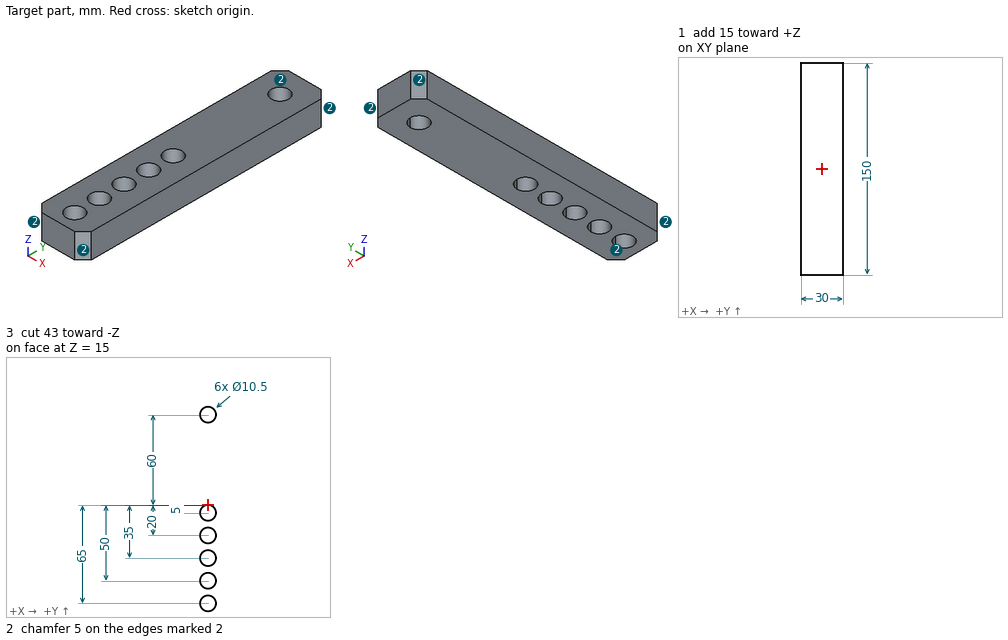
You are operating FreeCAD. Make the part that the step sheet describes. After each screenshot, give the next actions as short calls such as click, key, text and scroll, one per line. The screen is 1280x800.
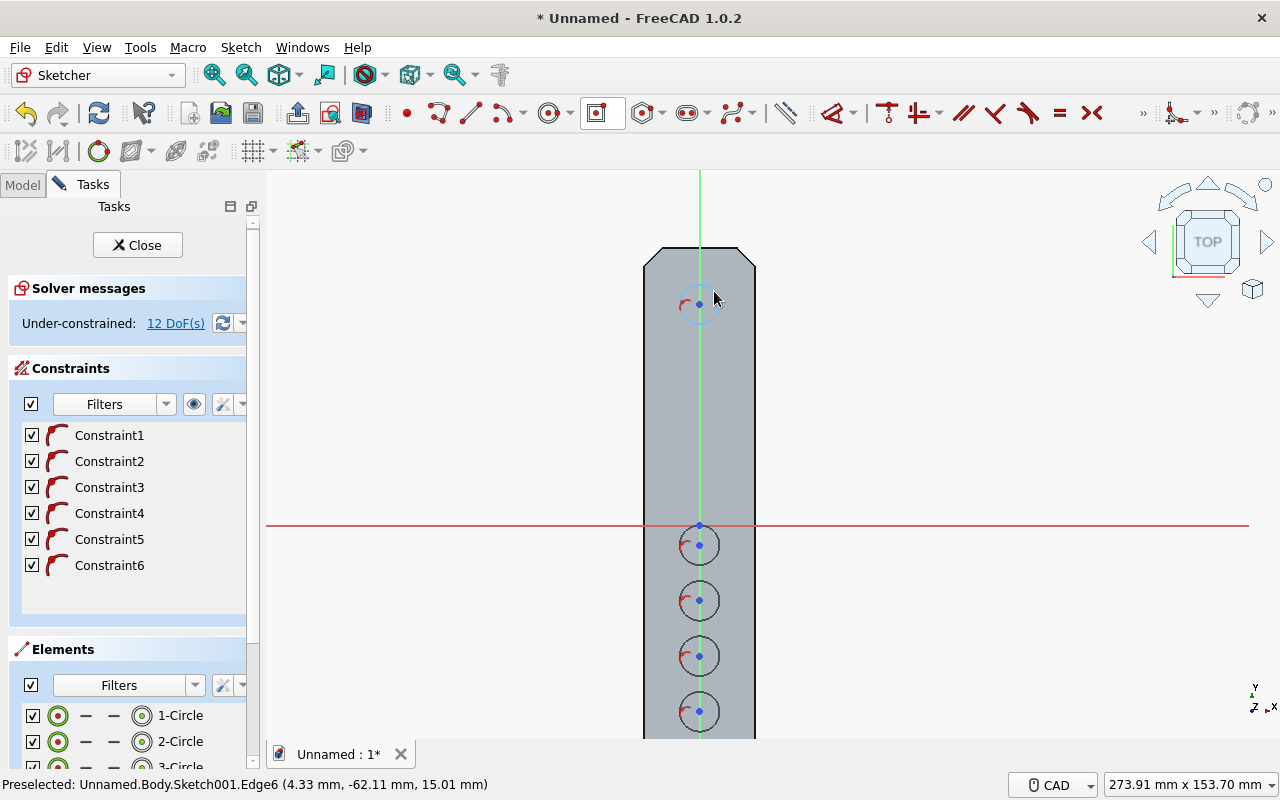
click(714, 290)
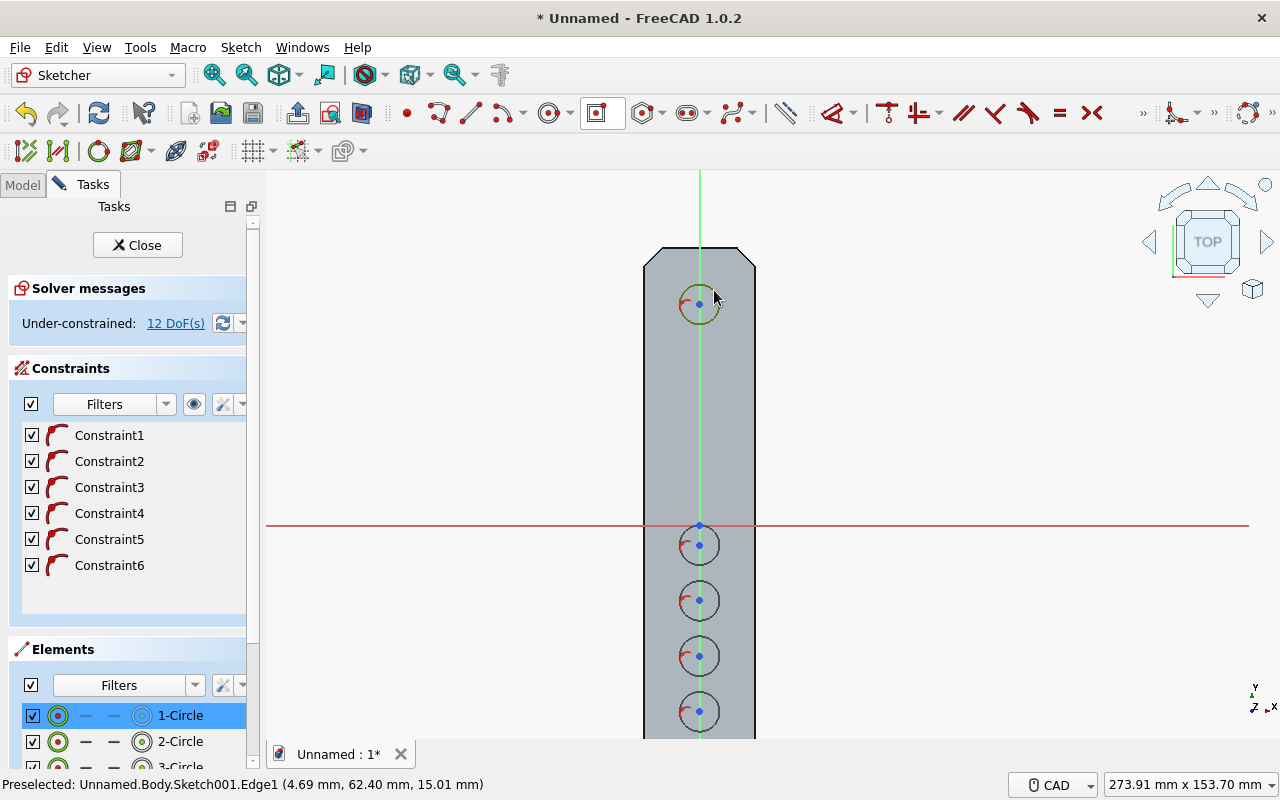
click(686, 559)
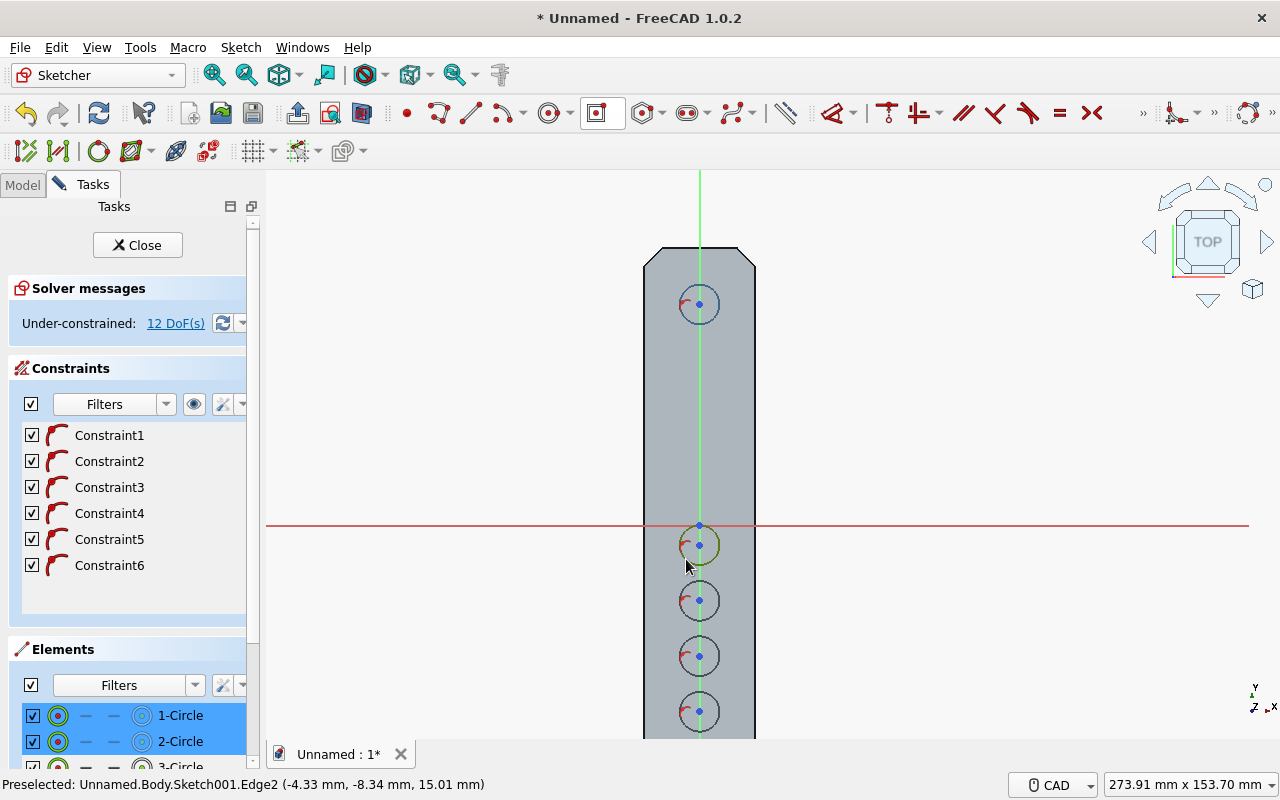
click(714, 587)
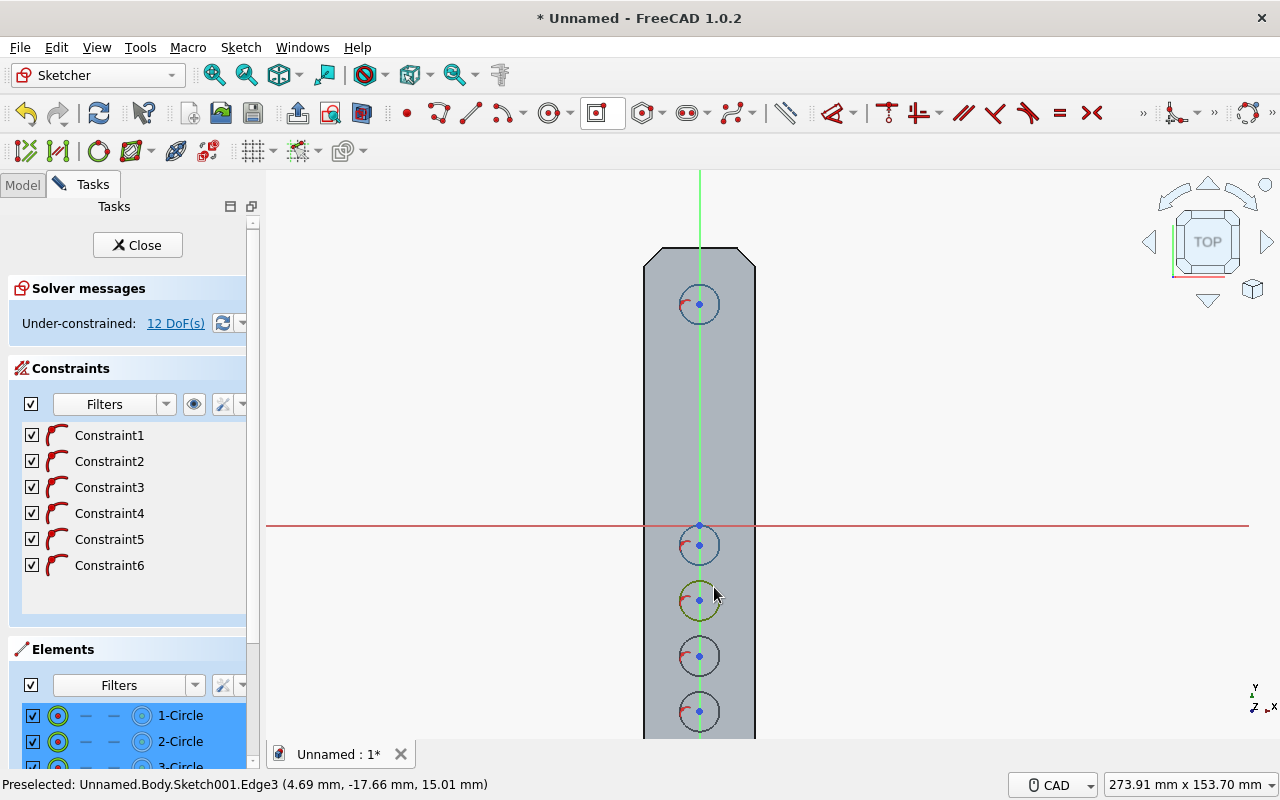
click(714, 642)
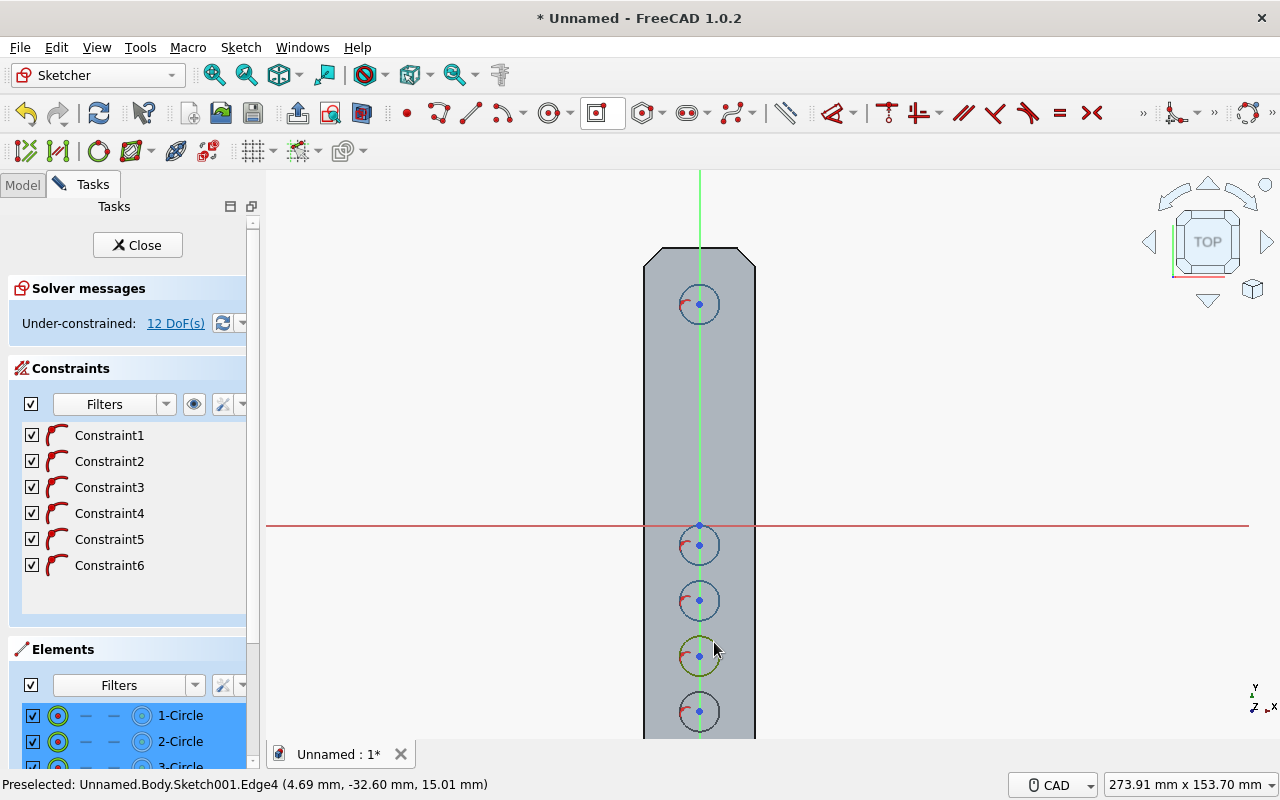
click(714, 698)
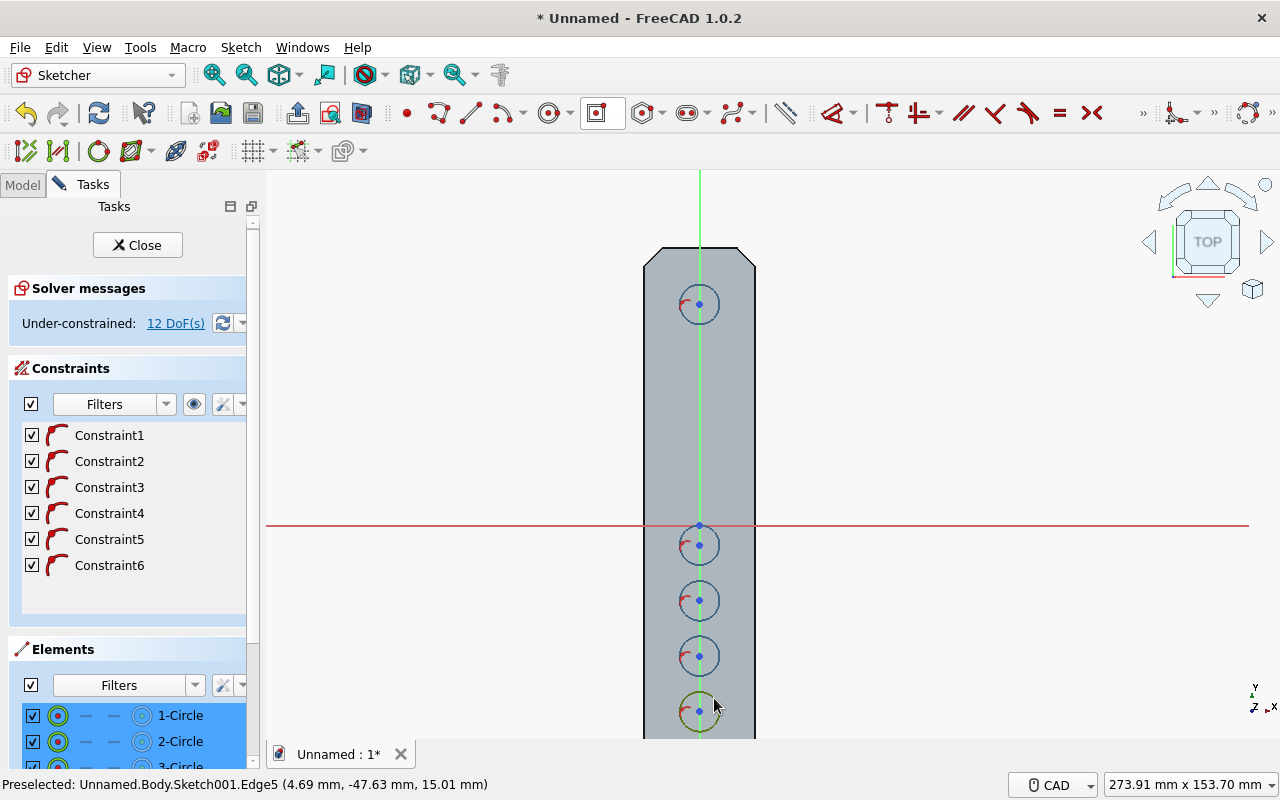
scroll(714, 290, down, 2)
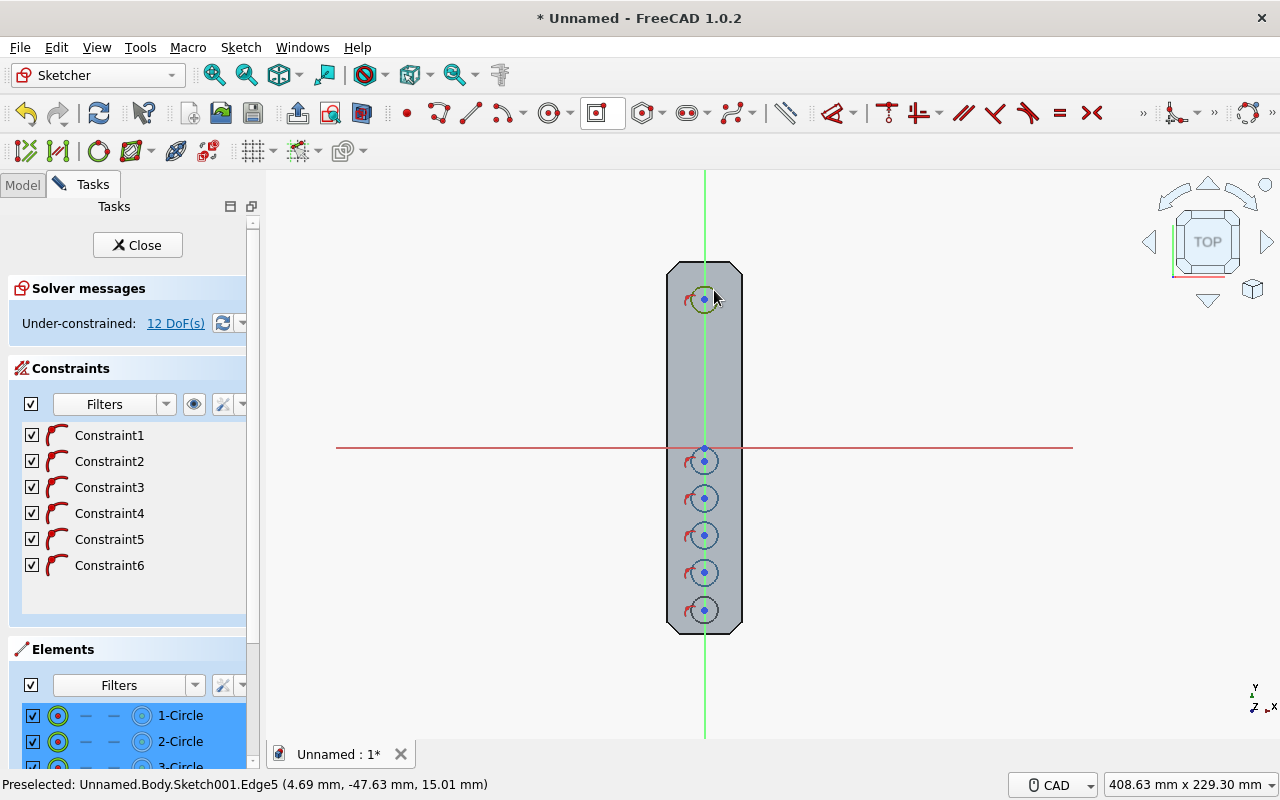
scroll(714, 601, up, 2)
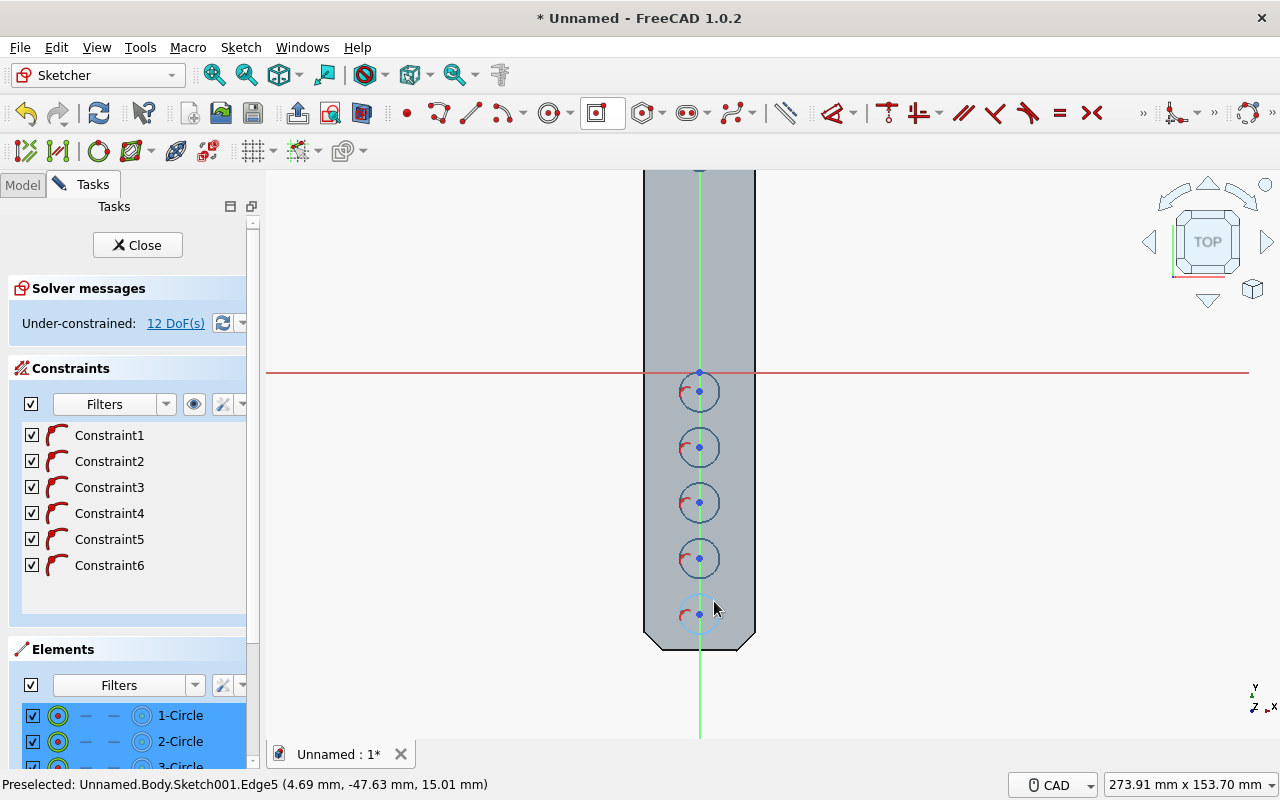
click(714, 600)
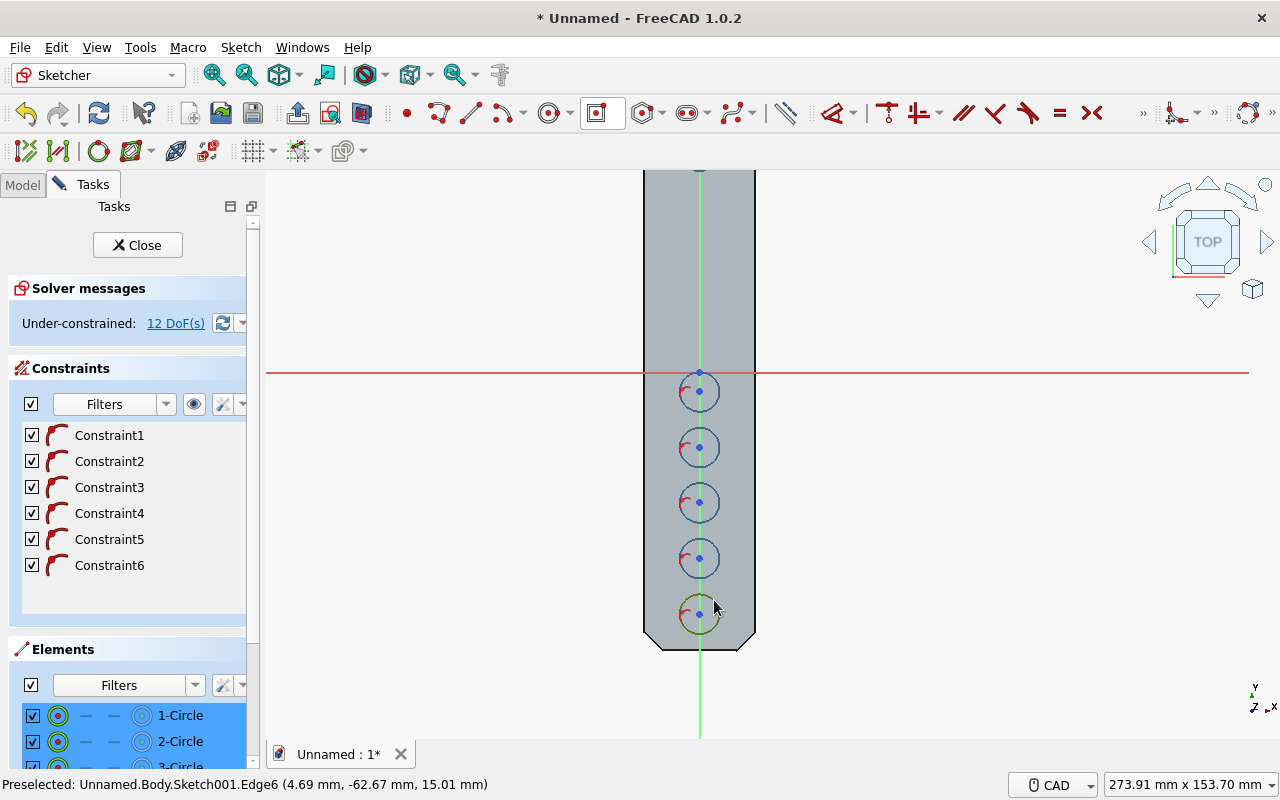
click(1060, 114)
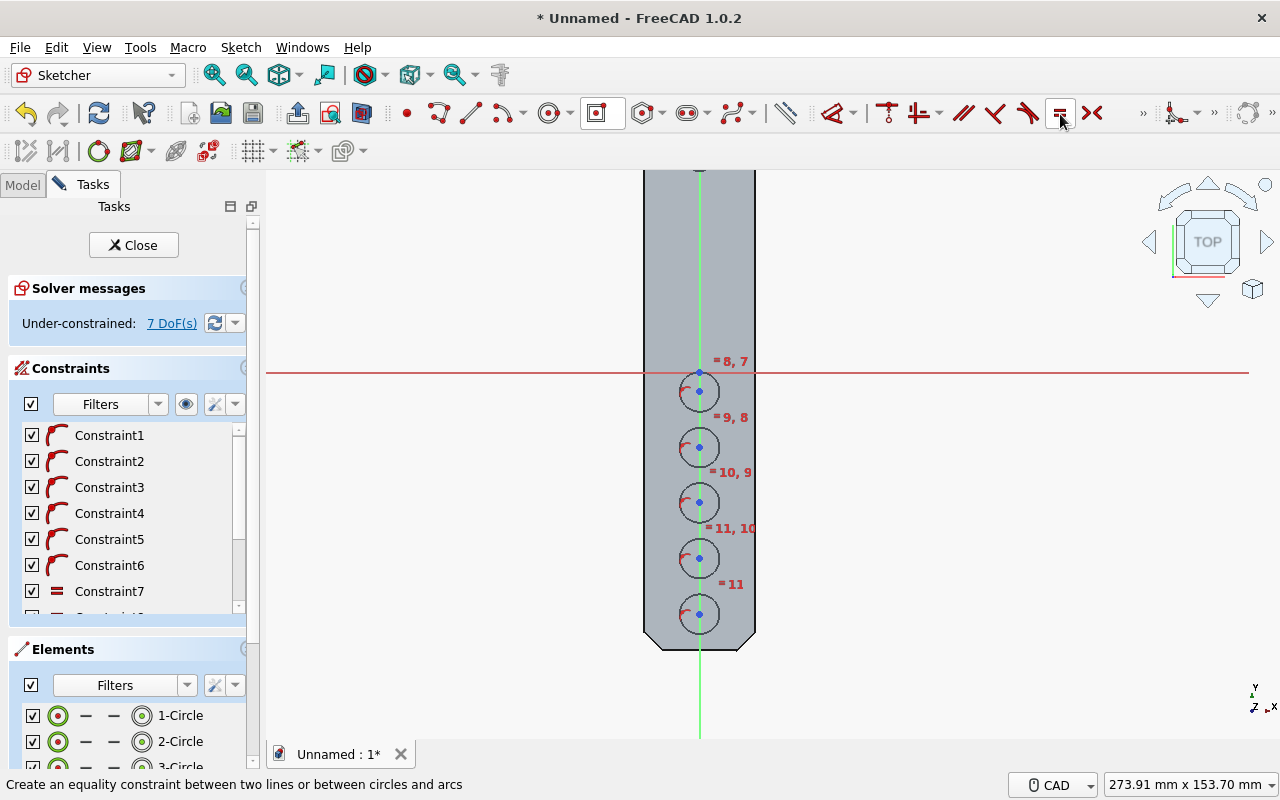
key(d)